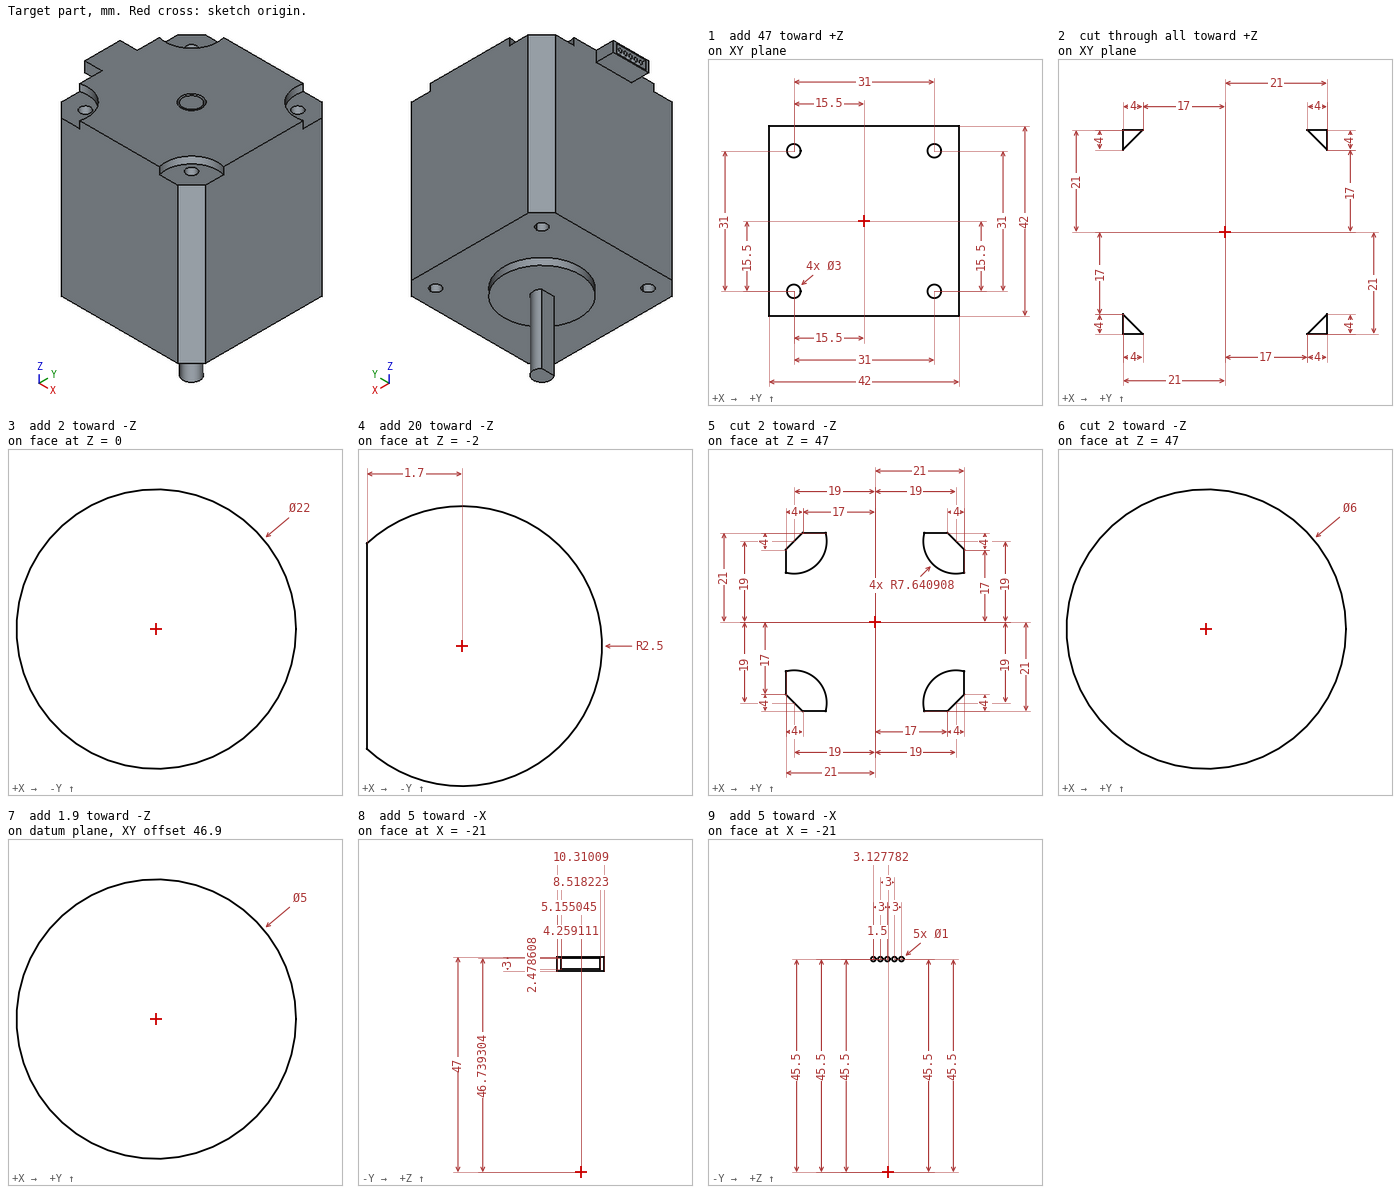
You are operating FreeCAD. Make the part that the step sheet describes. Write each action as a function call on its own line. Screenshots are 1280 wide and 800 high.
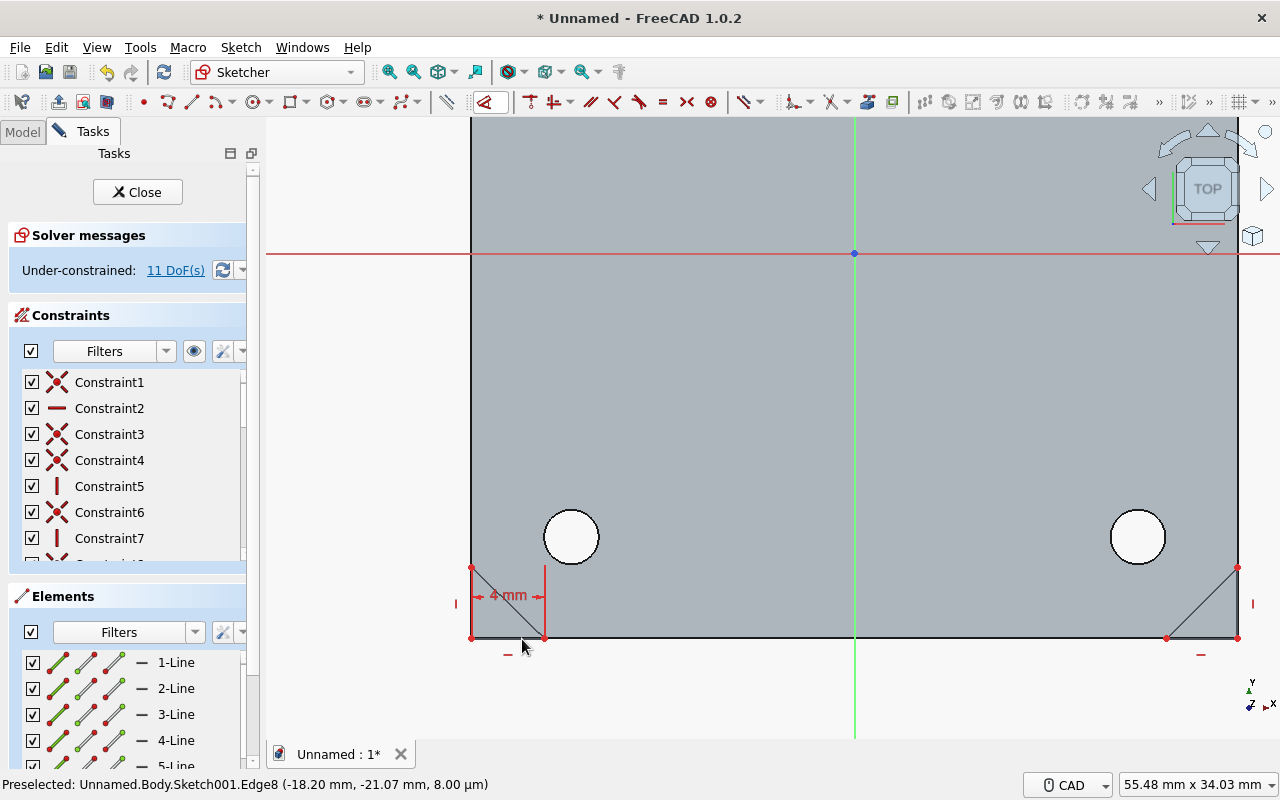
click(472, 617)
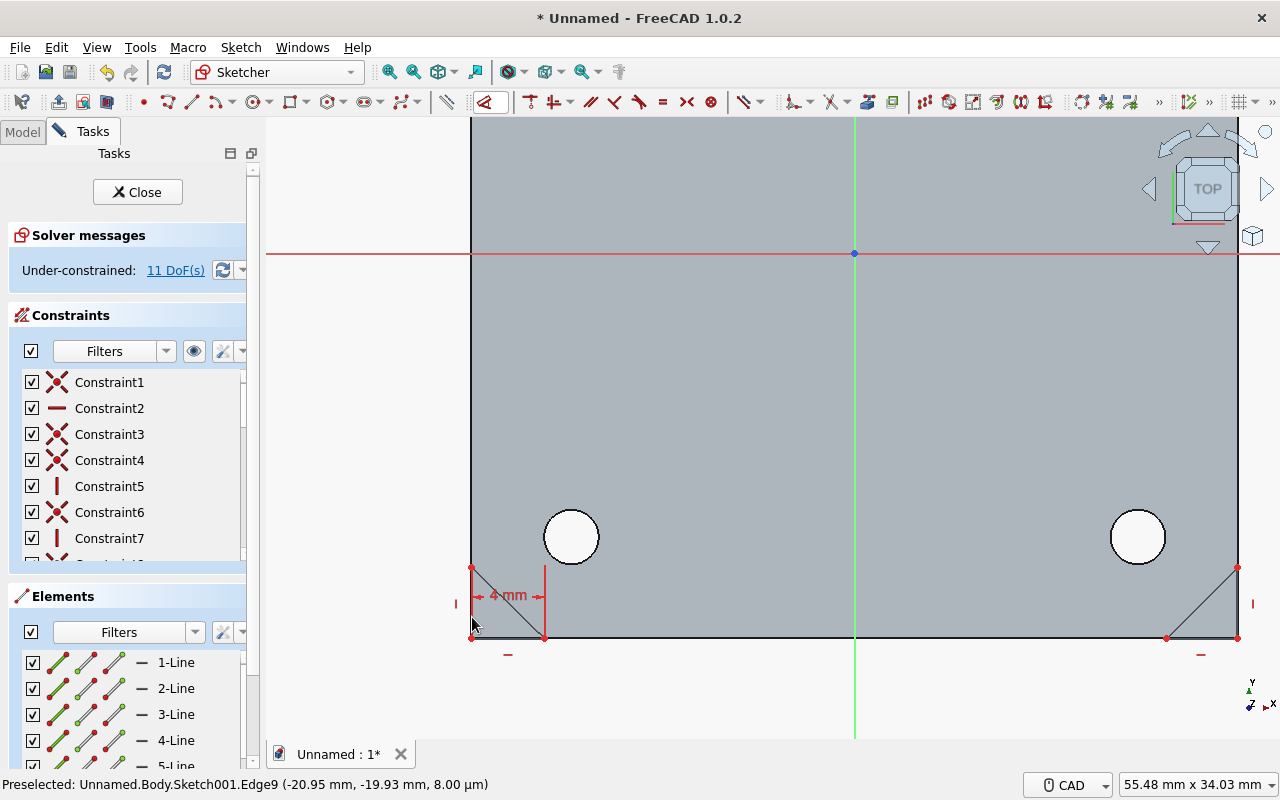
key(i)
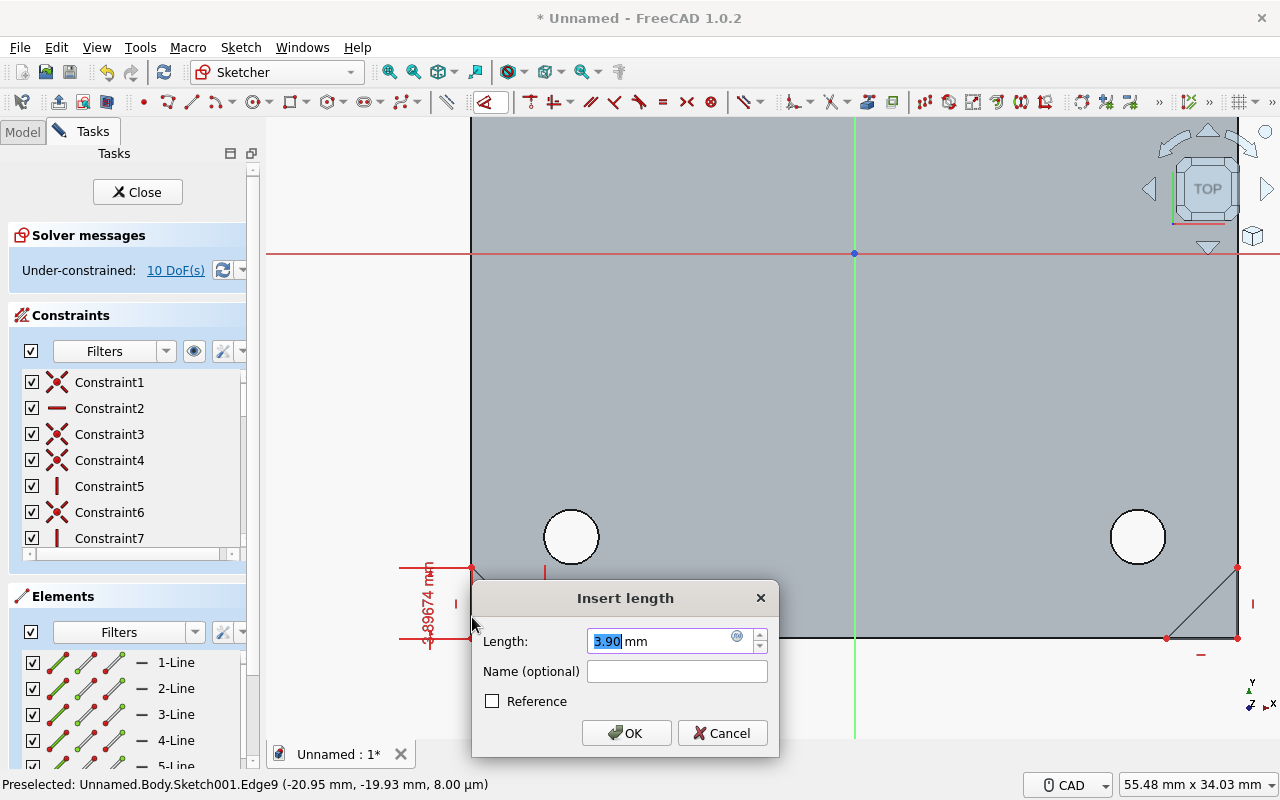
text(4)
key(Return)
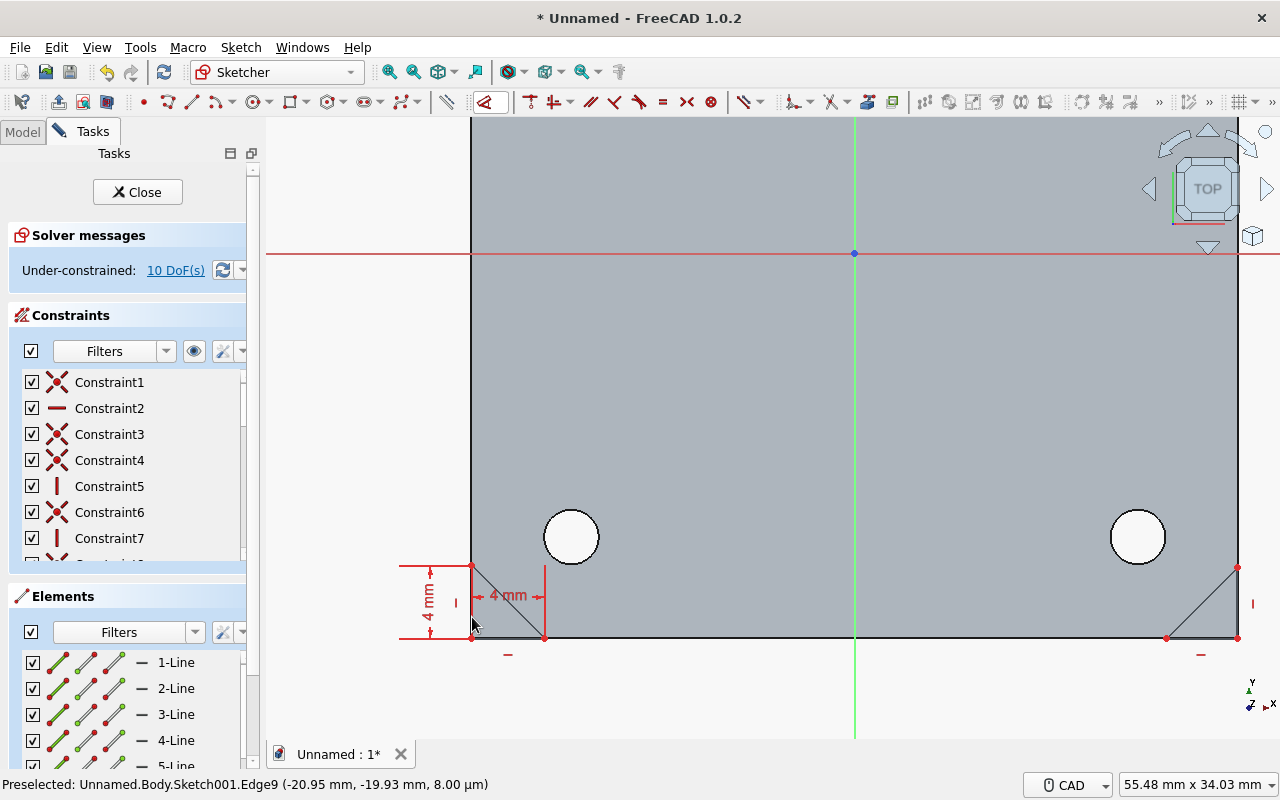
scroll(522, 640, down, 3)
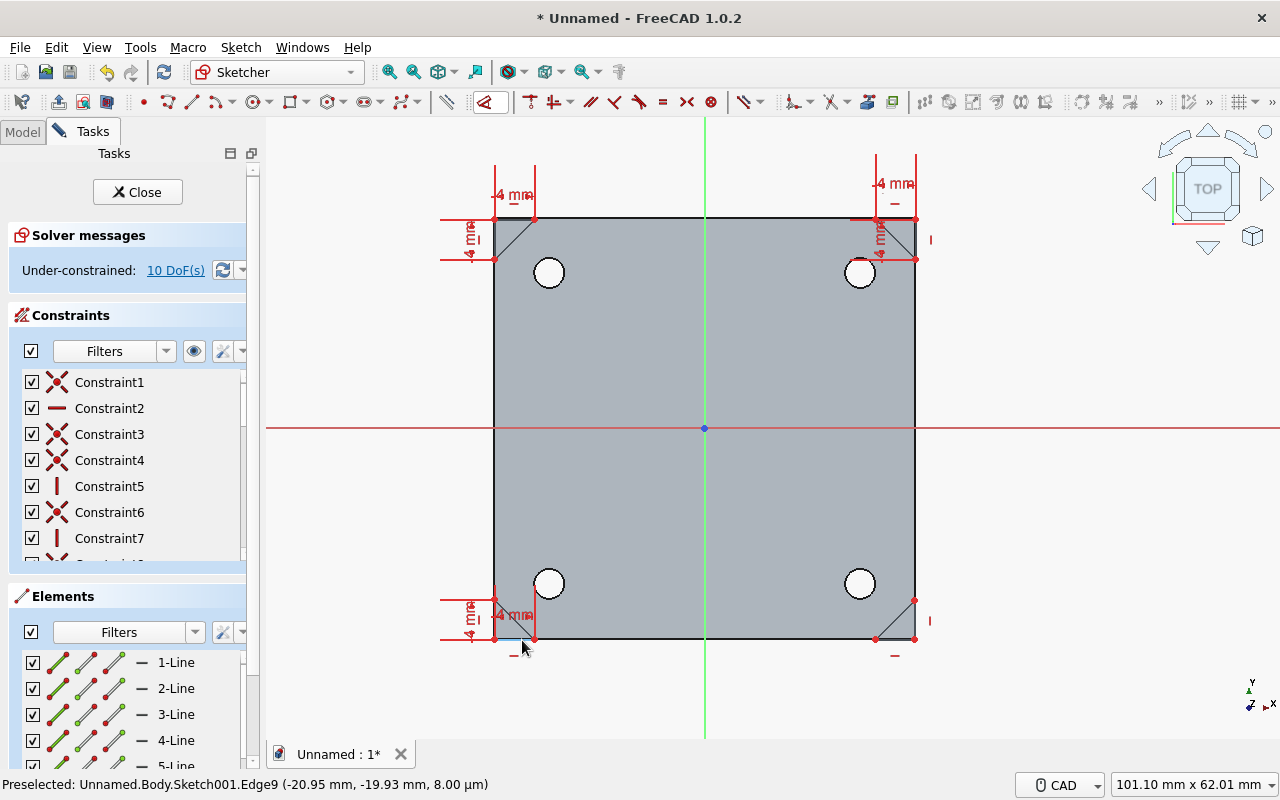
scroll(915, 612, up, 3)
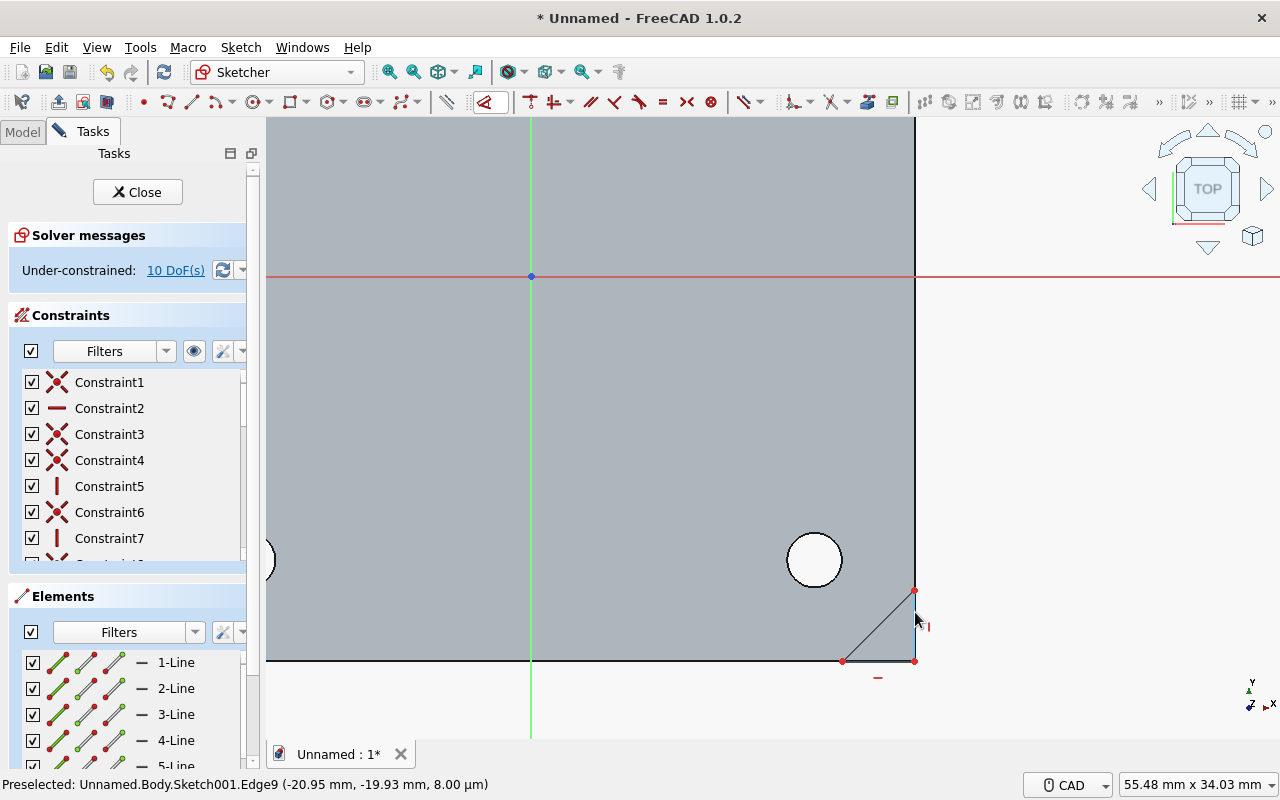
click(914, 612)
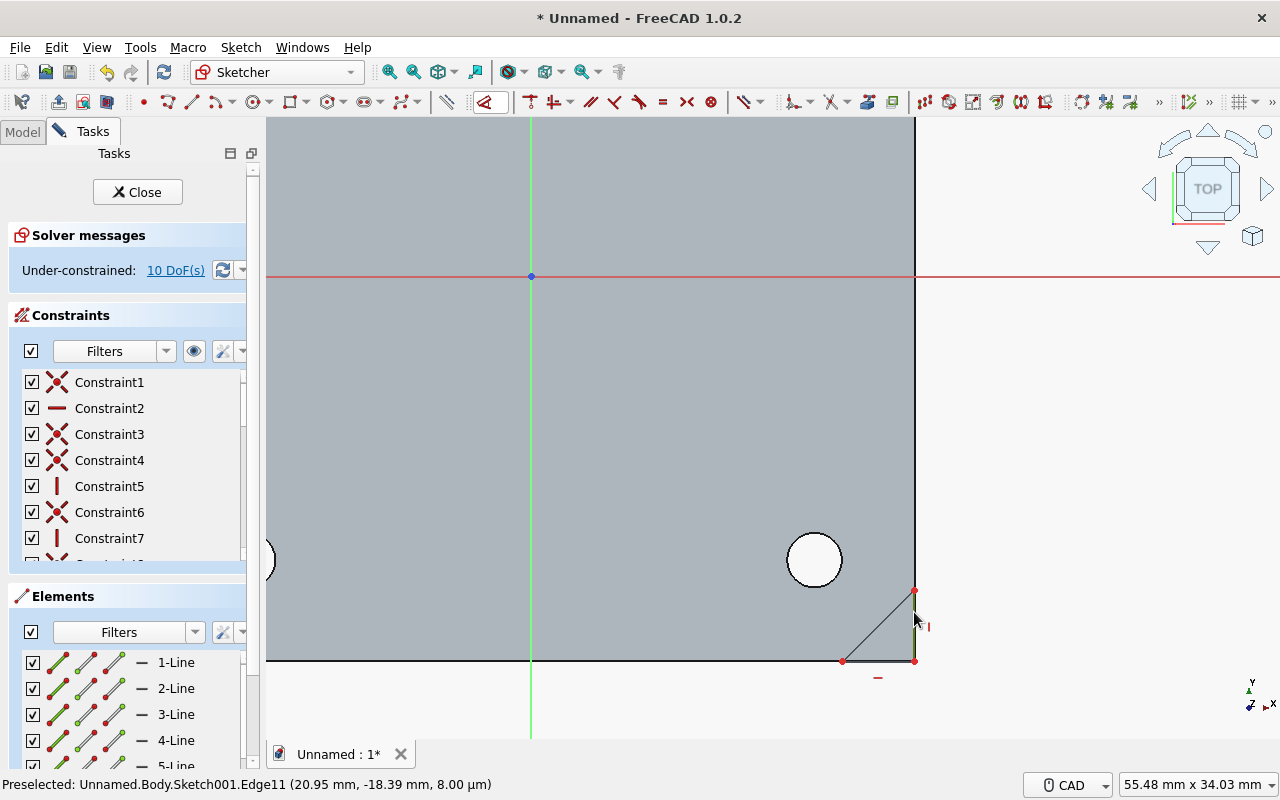
key(i)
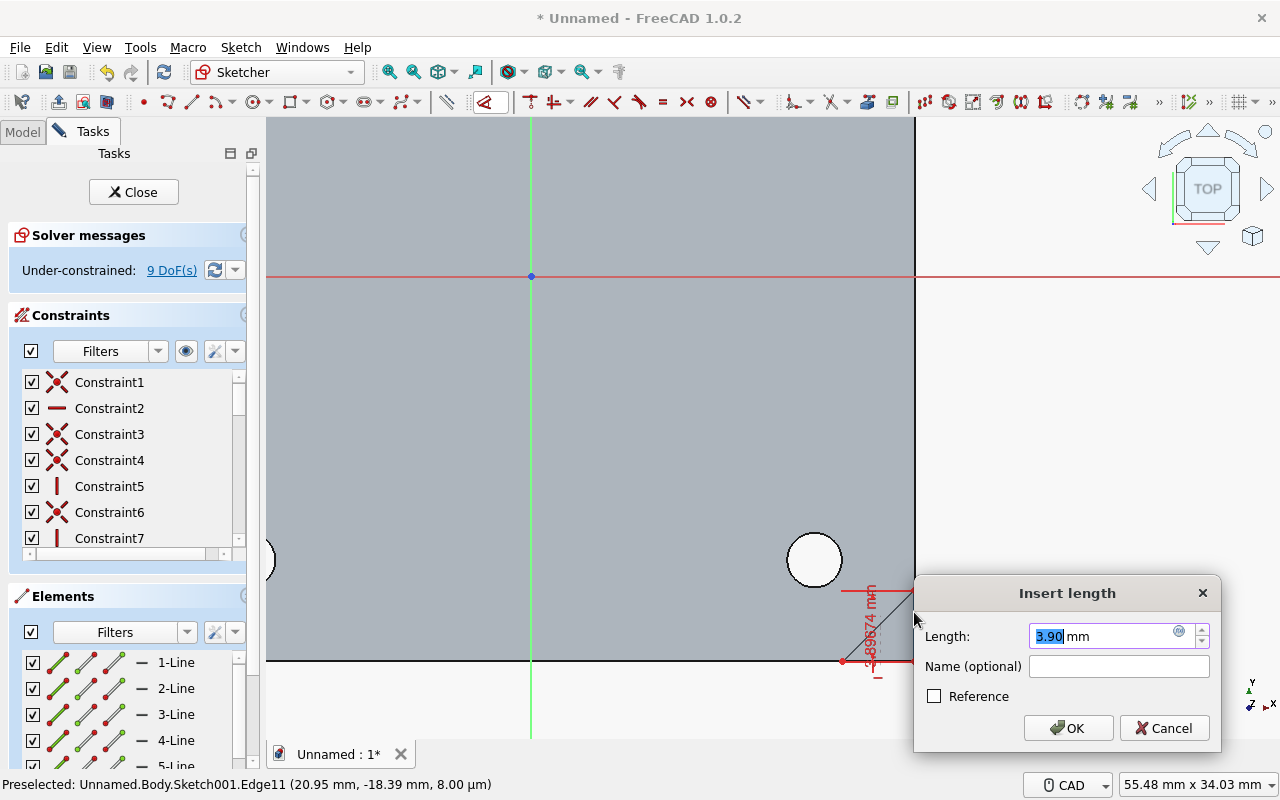
text(4)
key(Return)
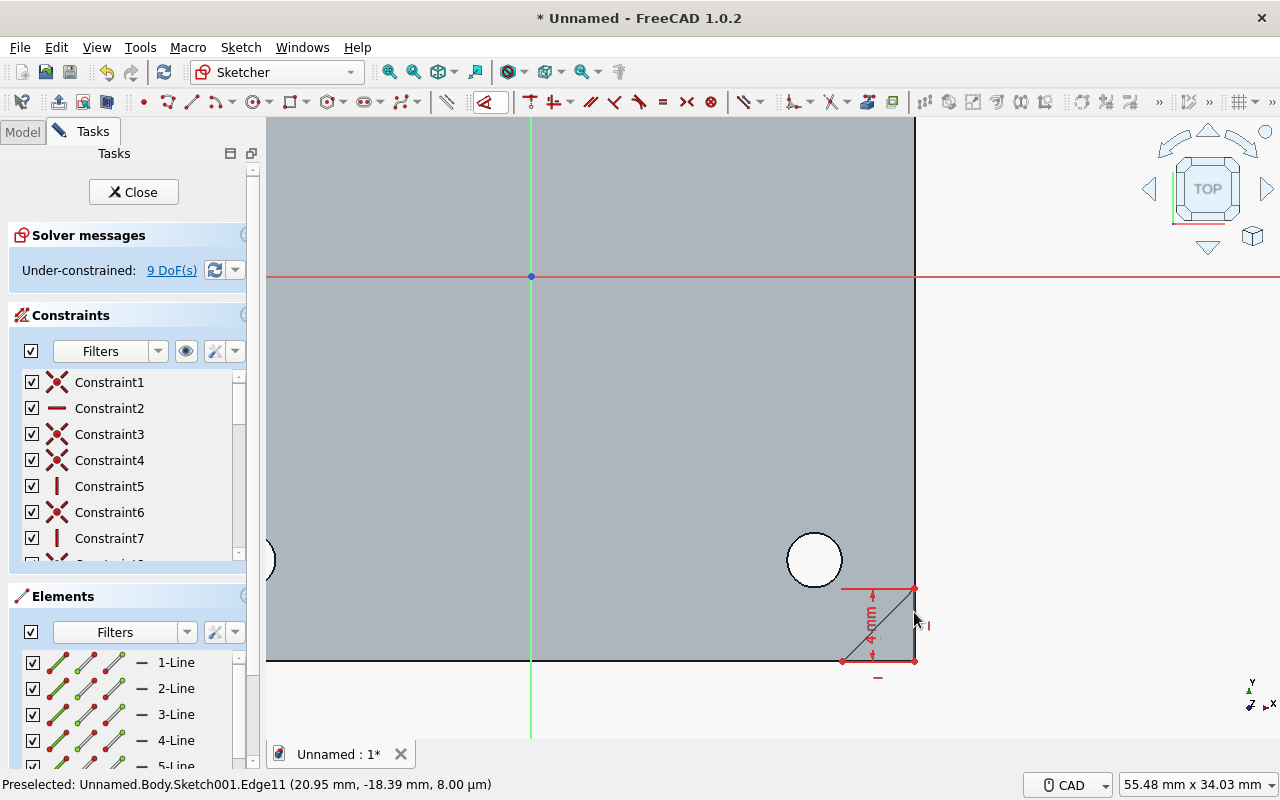
click(893, 662)